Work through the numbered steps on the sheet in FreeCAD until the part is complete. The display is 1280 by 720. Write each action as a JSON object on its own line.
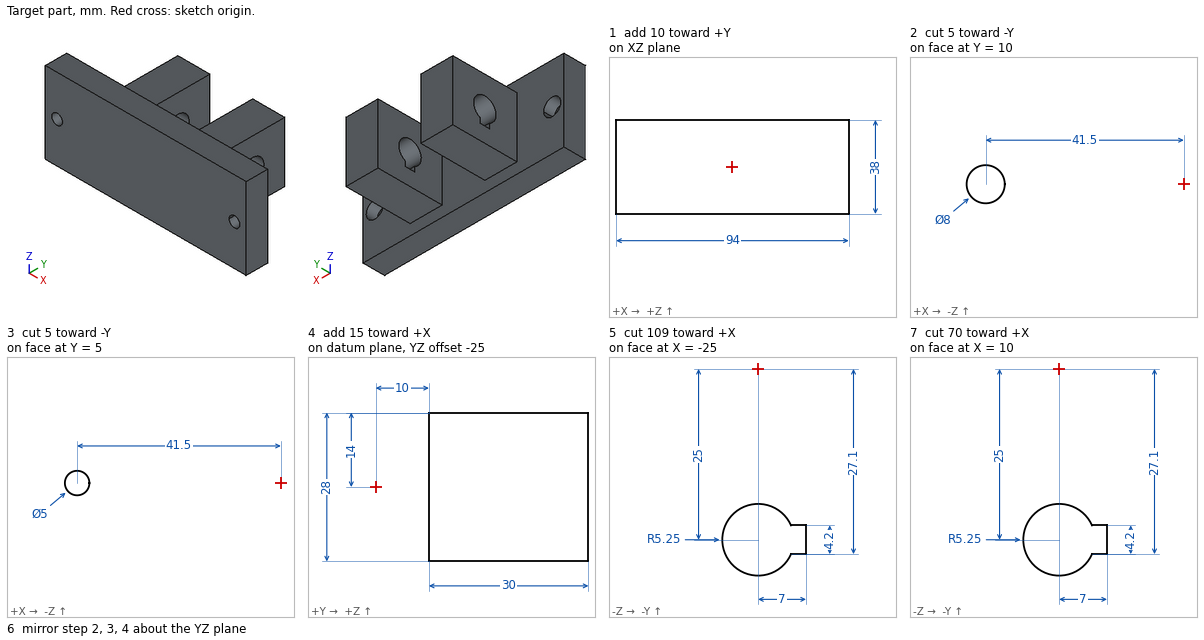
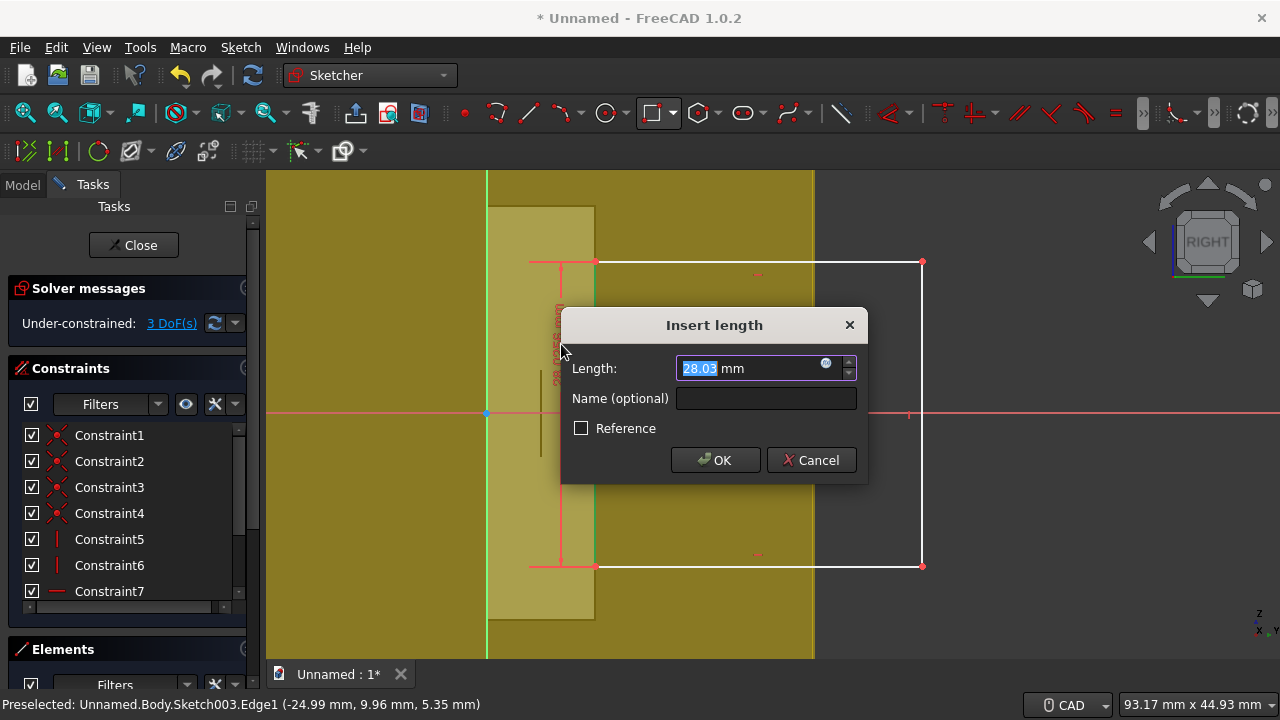
{"action": "type", "text": "28"}
{"action": "key", "text": "Return"}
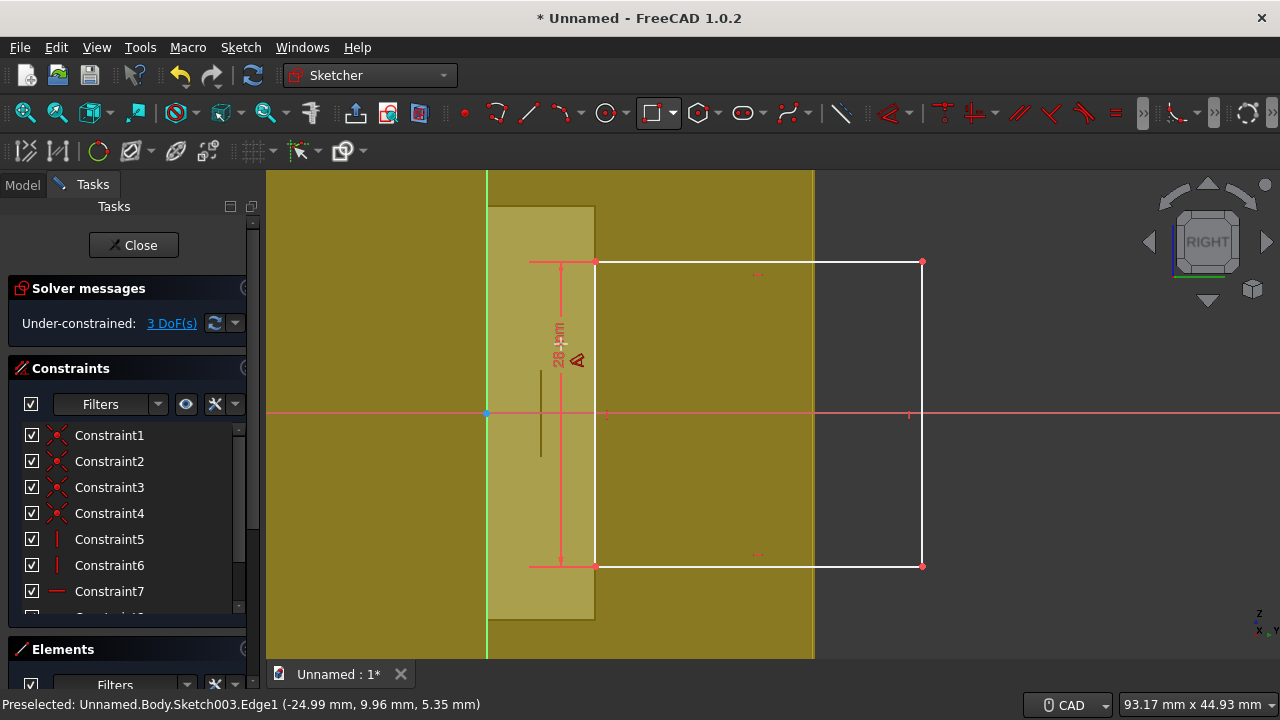
{"action": "left_click", "coordinate": [693, 567]}
{"action": "left_click", "coordinate": [759, 601]}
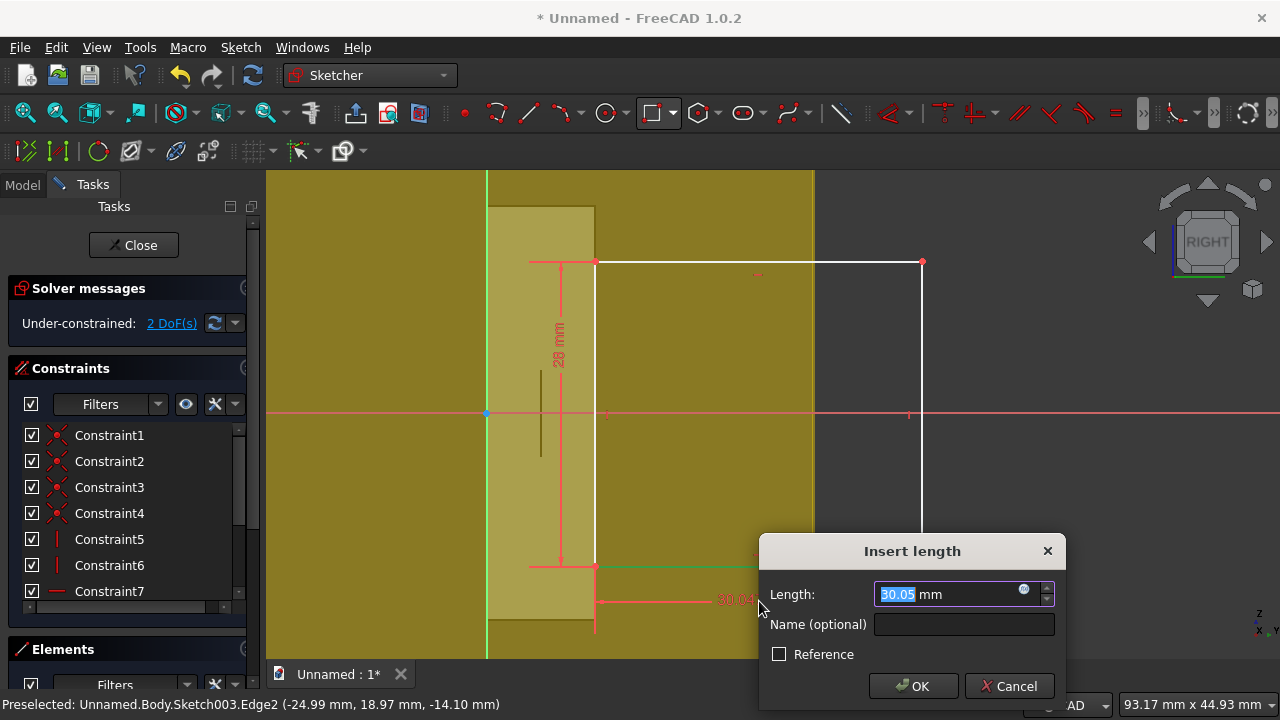
{"action": "type", "text": "30"}
{"action": "key", "text": "Return"}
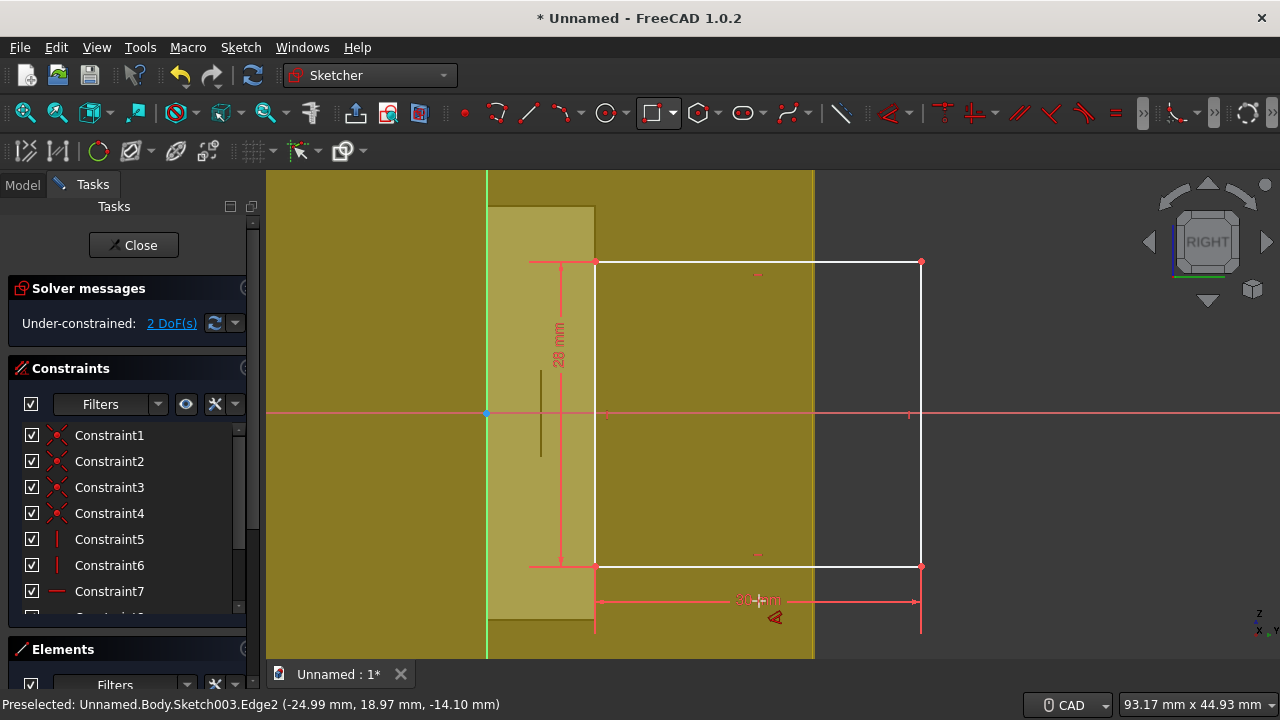
{"action": "left_click", "coordinate": [595, 262]}
{"action": "left_click", "coordinate": [541, 228]}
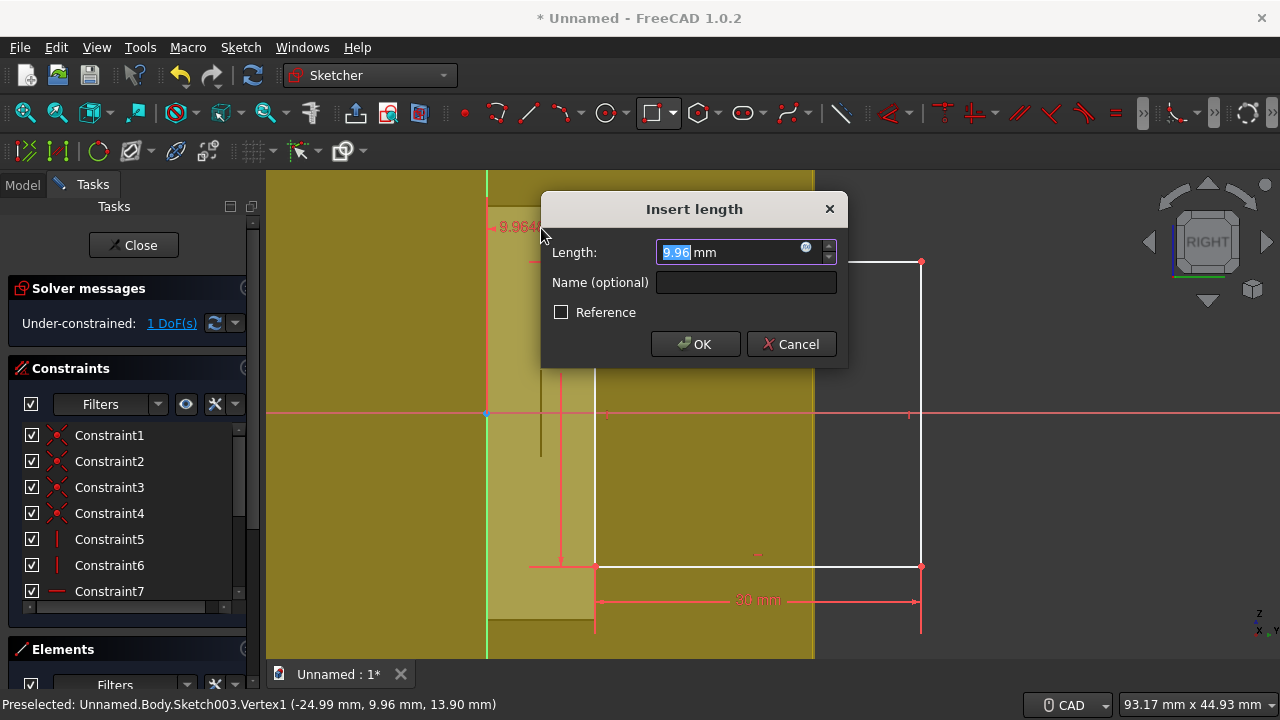
{"action": "type", "text": "10"}
{"action": "key", "text": "Return"}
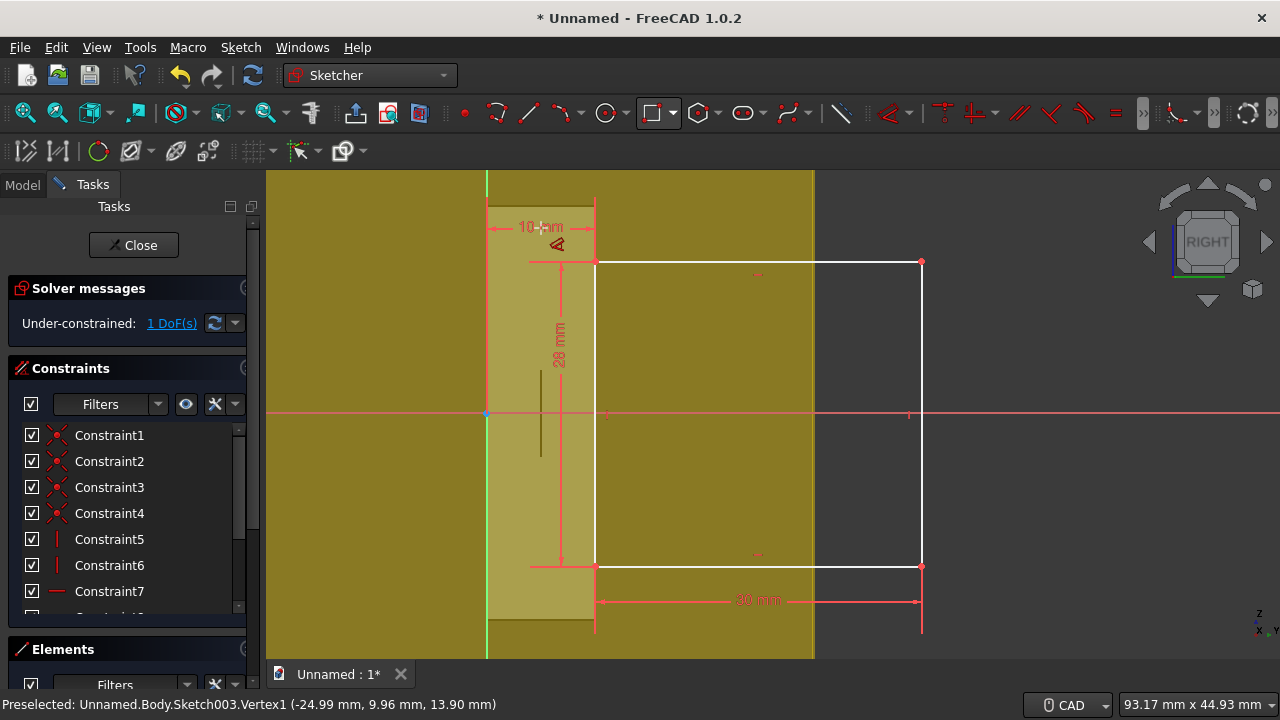
{"action": "left_click", "coordinate": [595, 262]}
{"action": "left_click", "coordinate": [453, 338]}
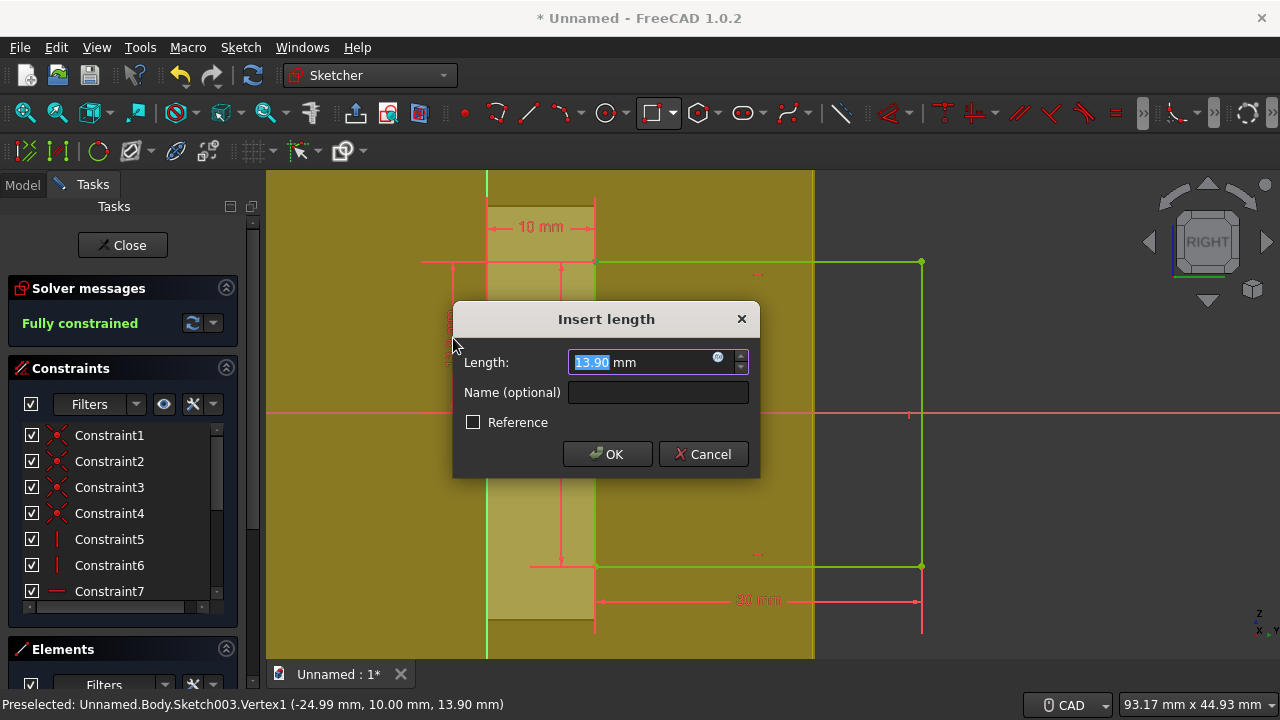
{"action": "type", "text": "14"}
{"action": "key", "text": "Return"}
{"action": "key", "text": "Escape"}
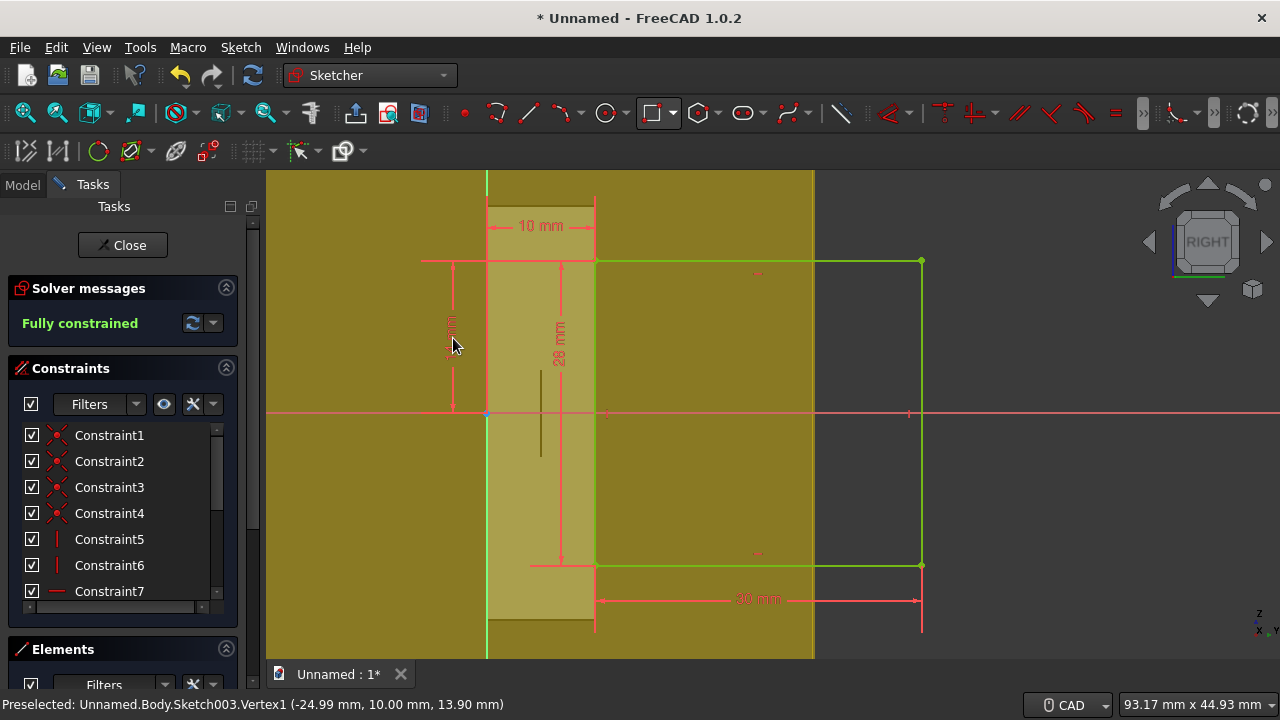
{"action": "left_click", "coordinate": [123, 245]}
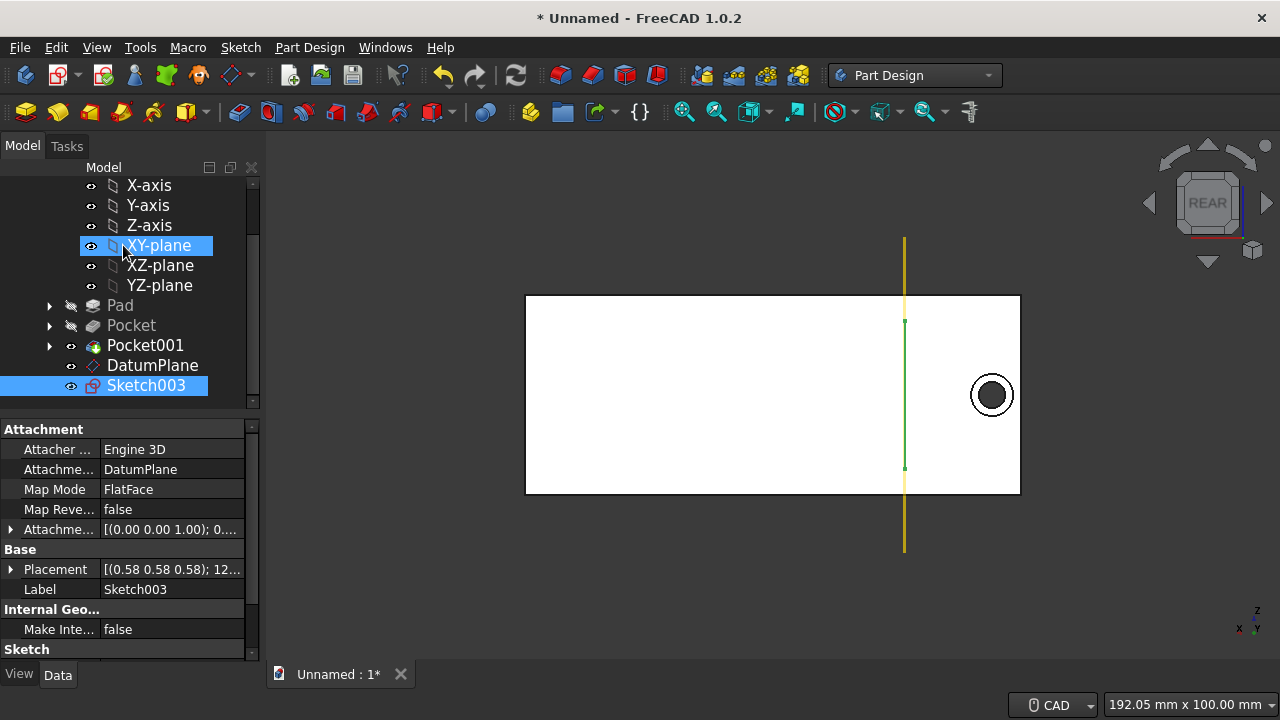
{"action": "left_click", "coordinate": [26, 112]}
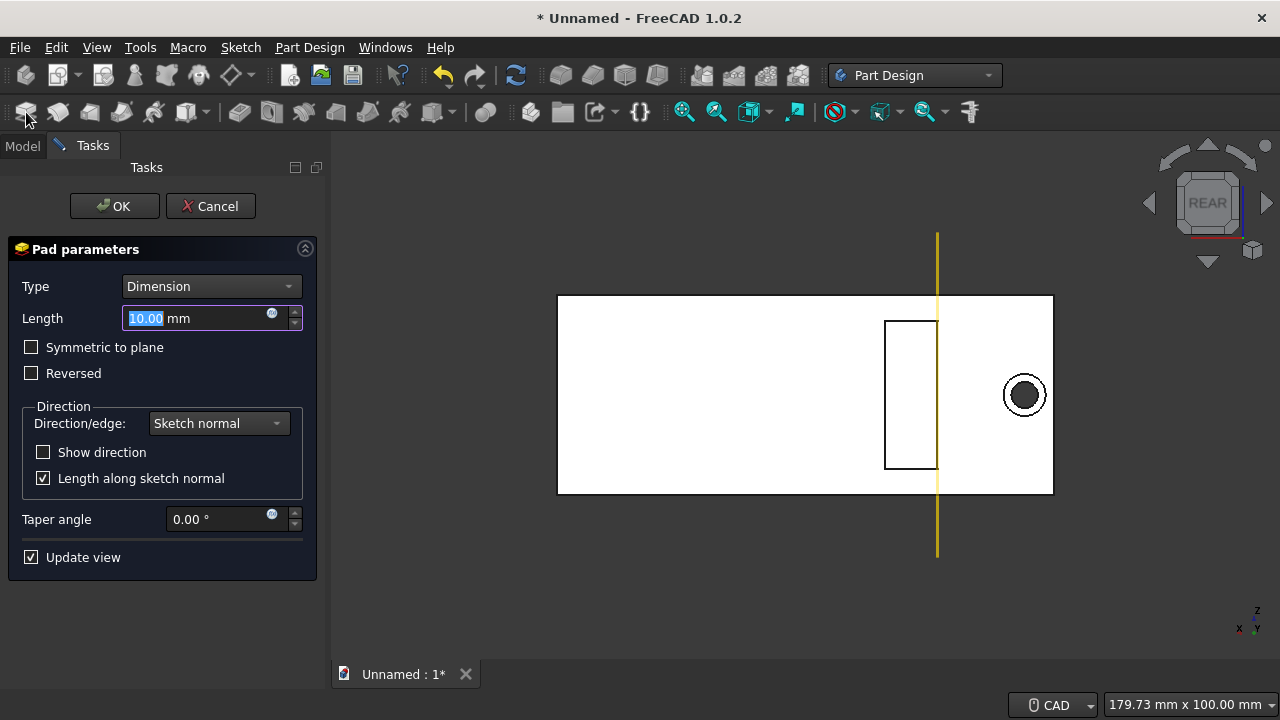
{"action": "type", "text": "15"}
{"action": "key", "text": "Tab"}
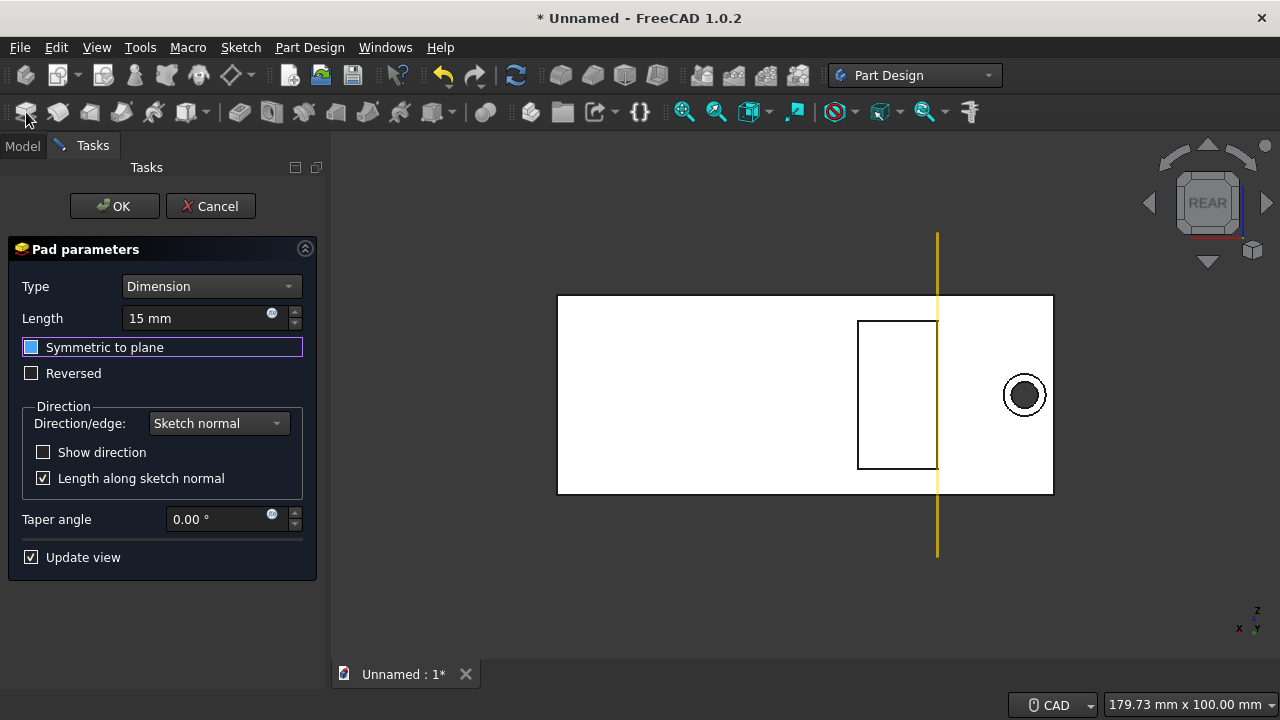
{"action": "left_click", "coordinate": [115, 206]}